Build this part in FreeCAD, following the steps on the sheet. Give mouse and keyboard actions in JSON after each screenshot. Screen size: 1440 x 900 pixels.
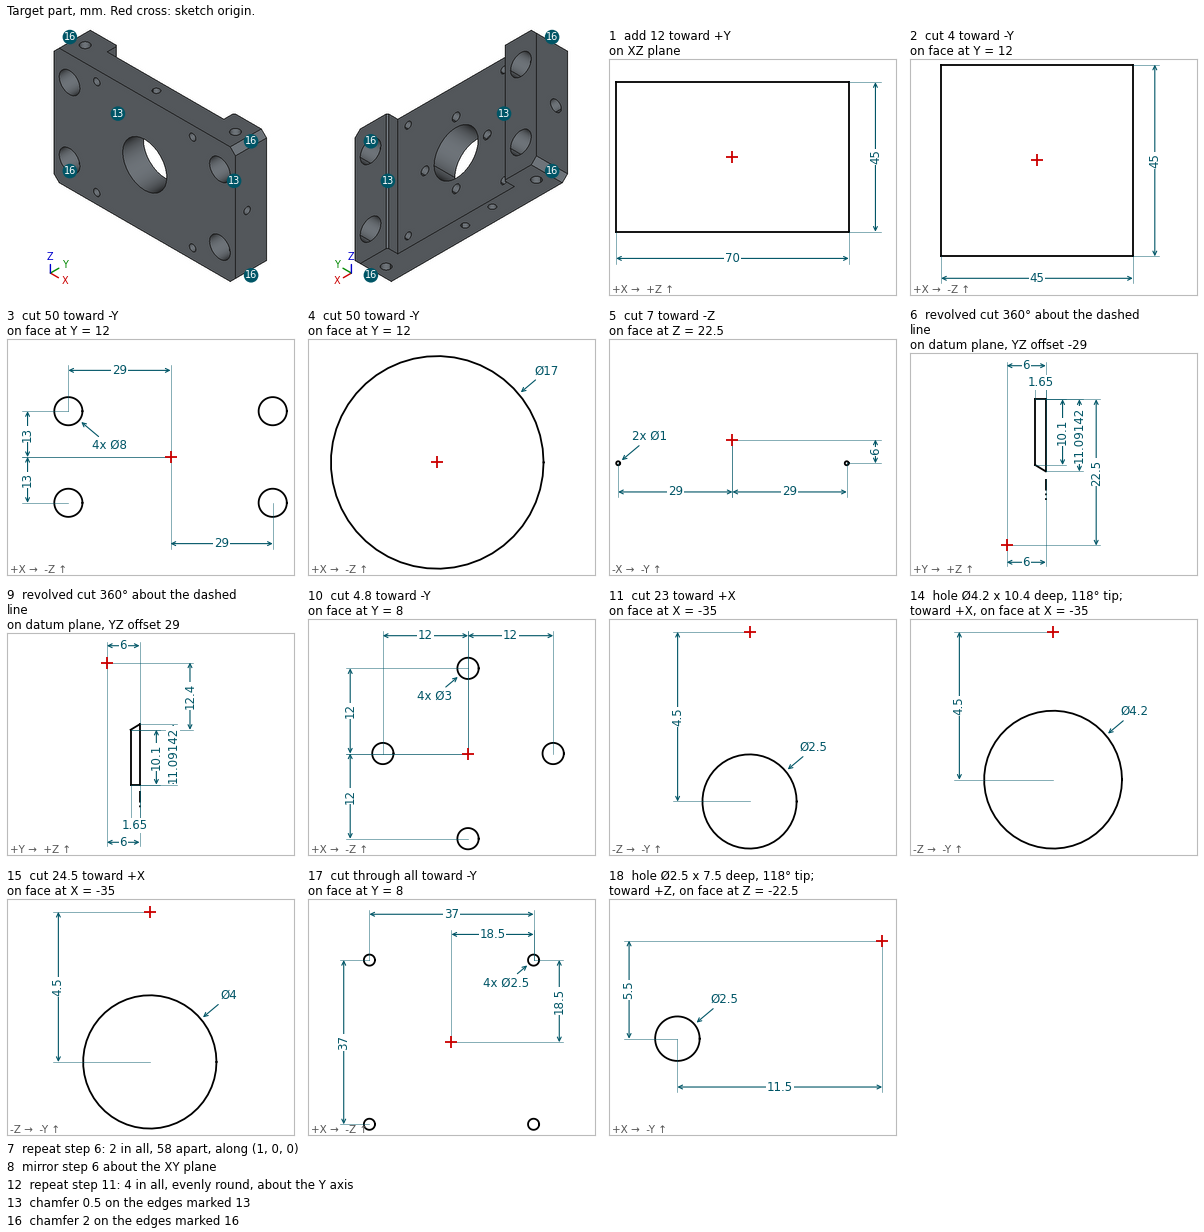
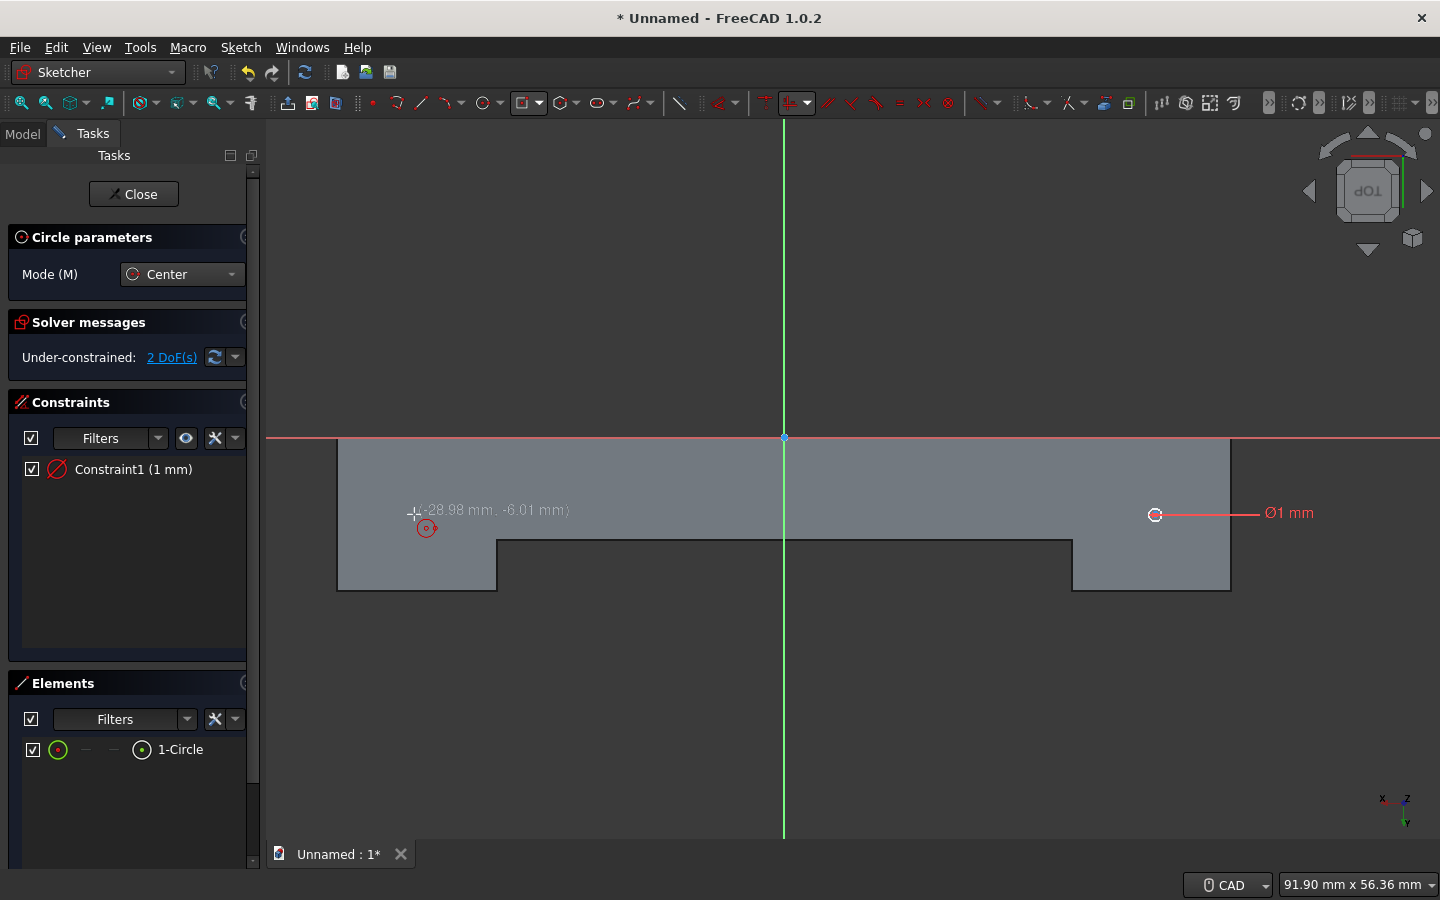
{"action": "left_click", "coordinate": [414, 514]}
{"action": "mouse_move", "coordinate": [418, 510]}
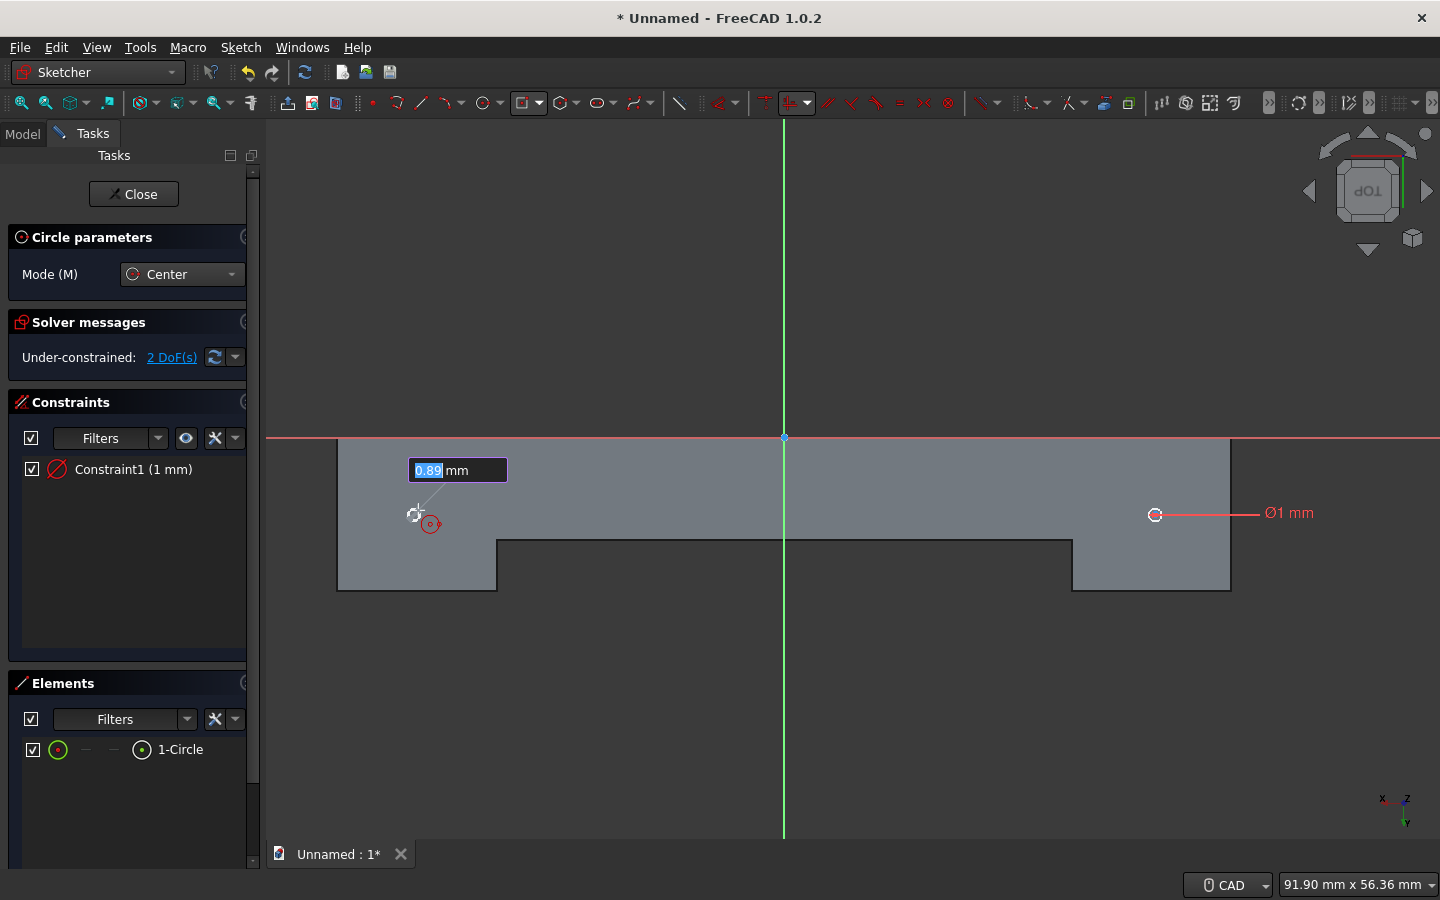
{"action": "type", "text": "1"}
{"action": "key", "text": "Return"}
{"action": "key", "text": "Escape"}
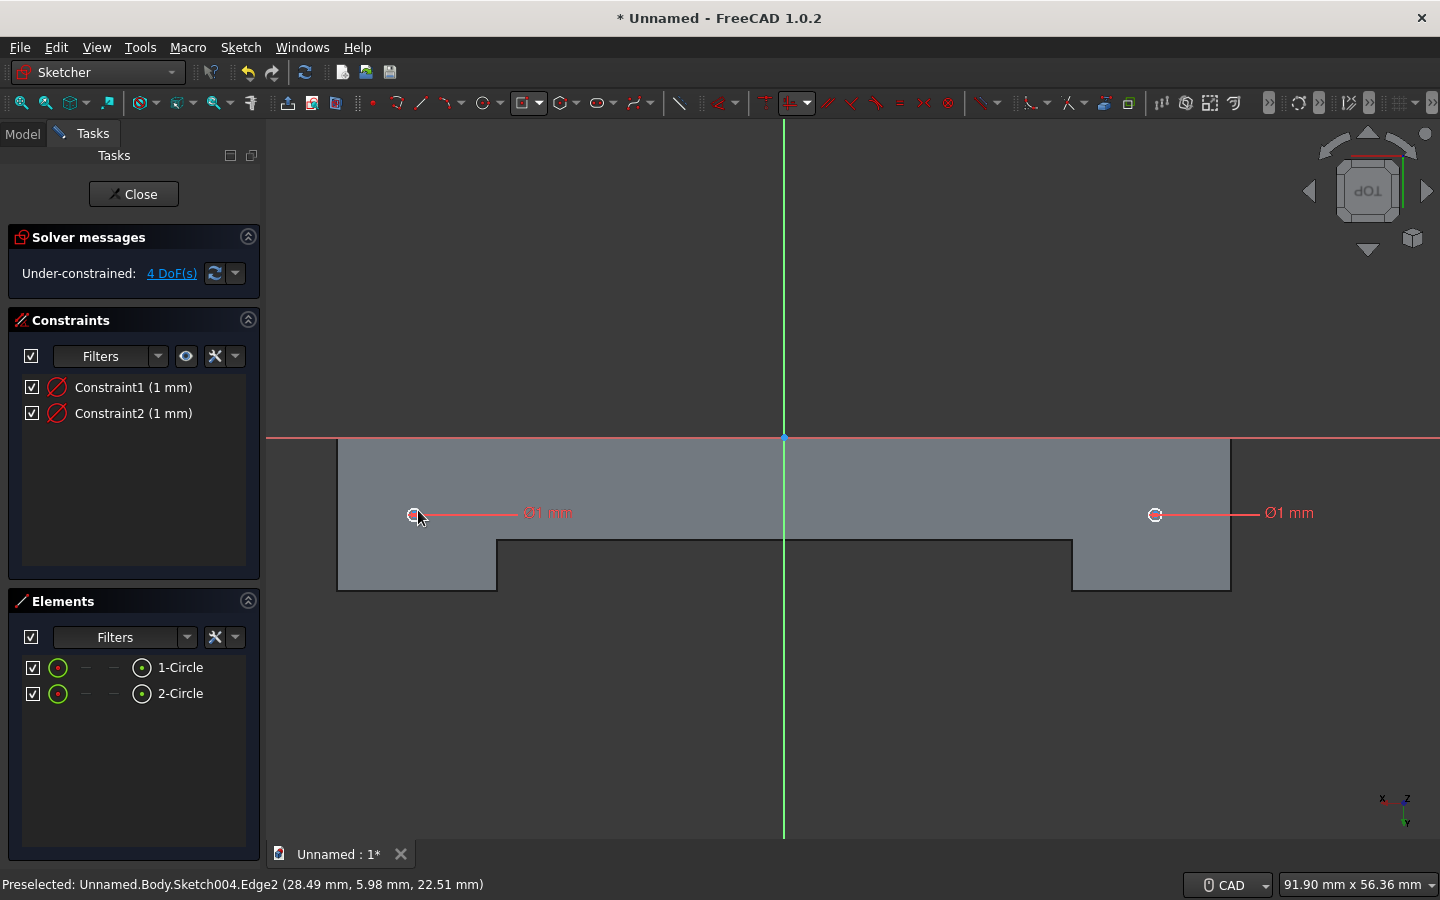
{"action": "left_click", "coordinate": [1155, 515]}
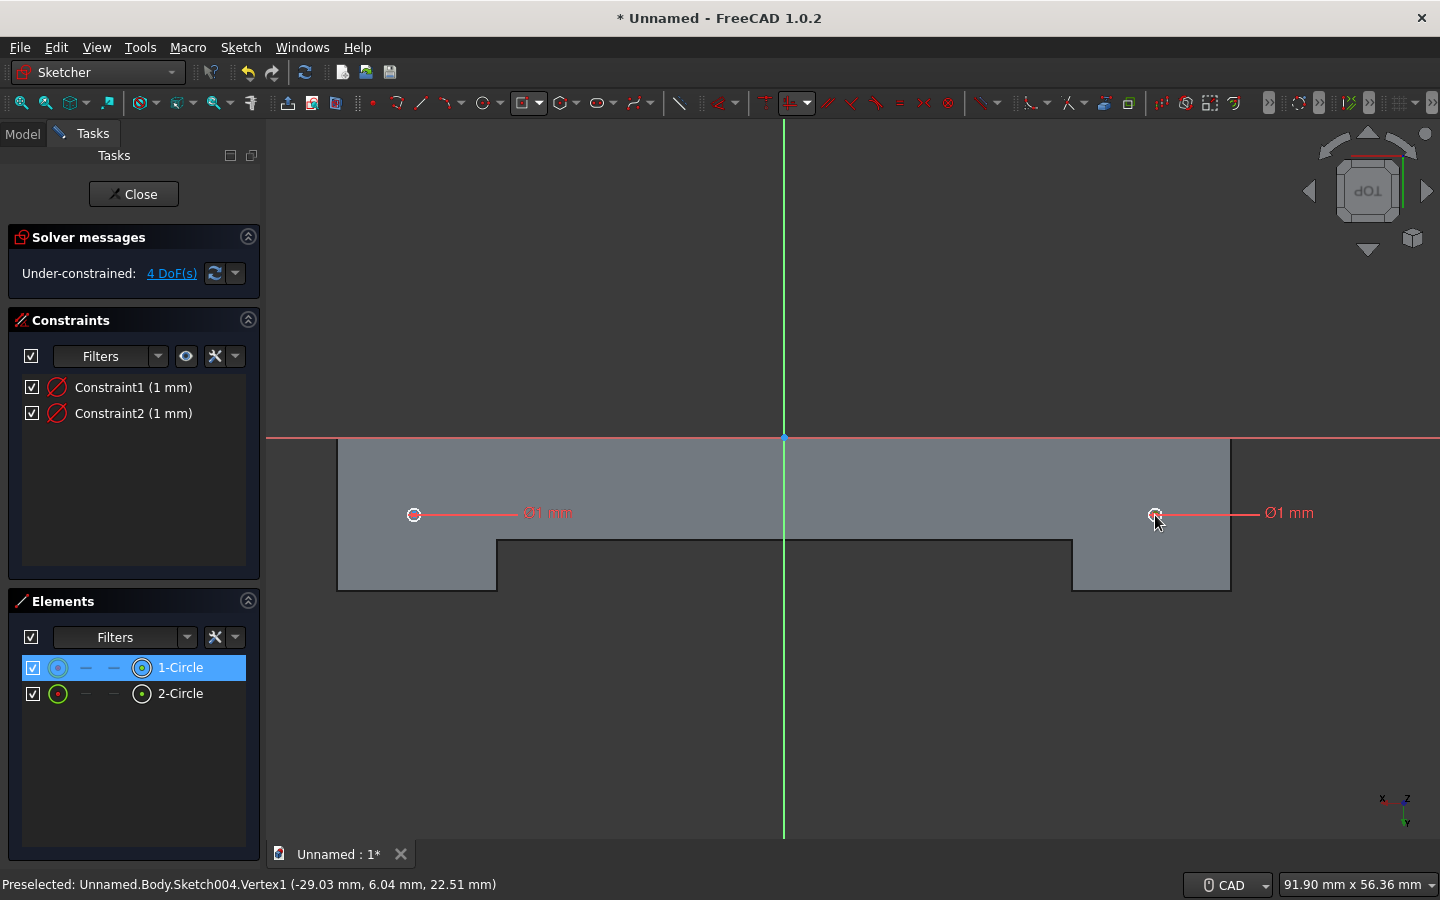
{"action": "left_click", "coordinate": [414, 515]}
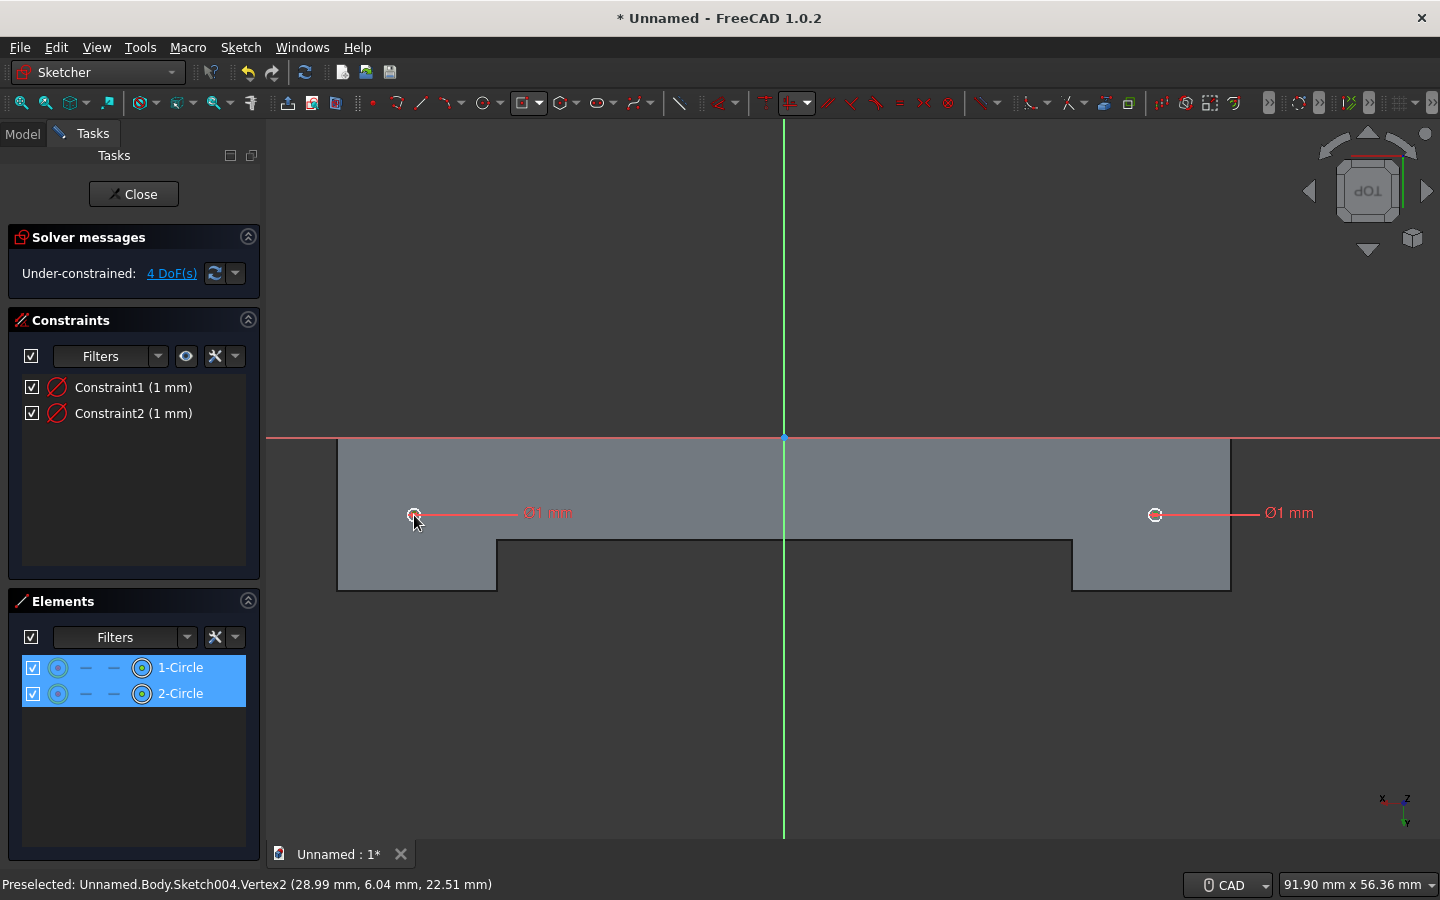
{"action": "left_click", "coordinate": [810, 104]}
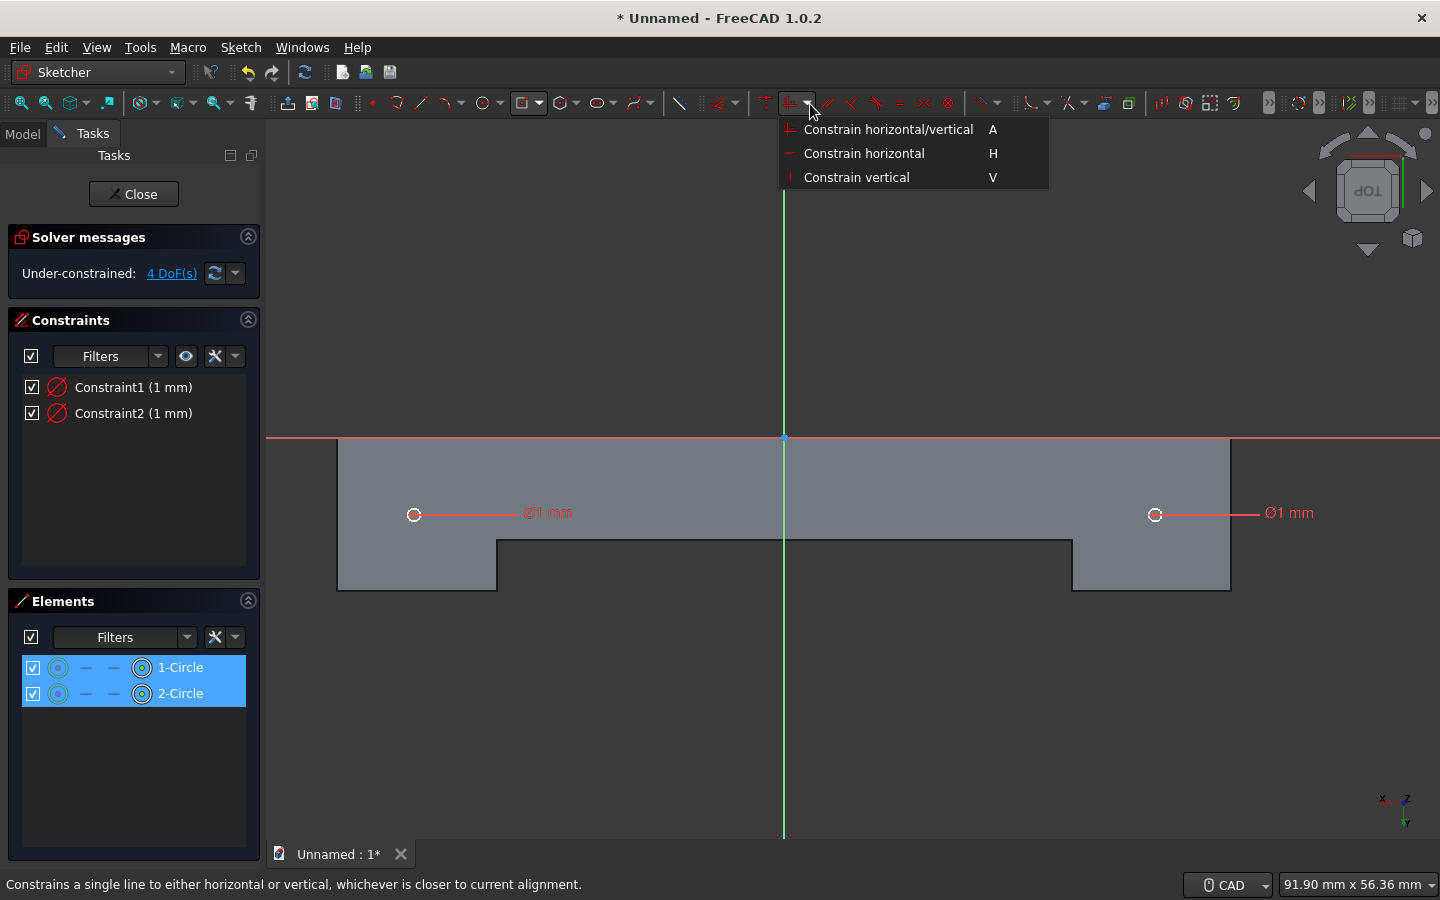
{"action": "left_click", "coordinate": [914, 153]}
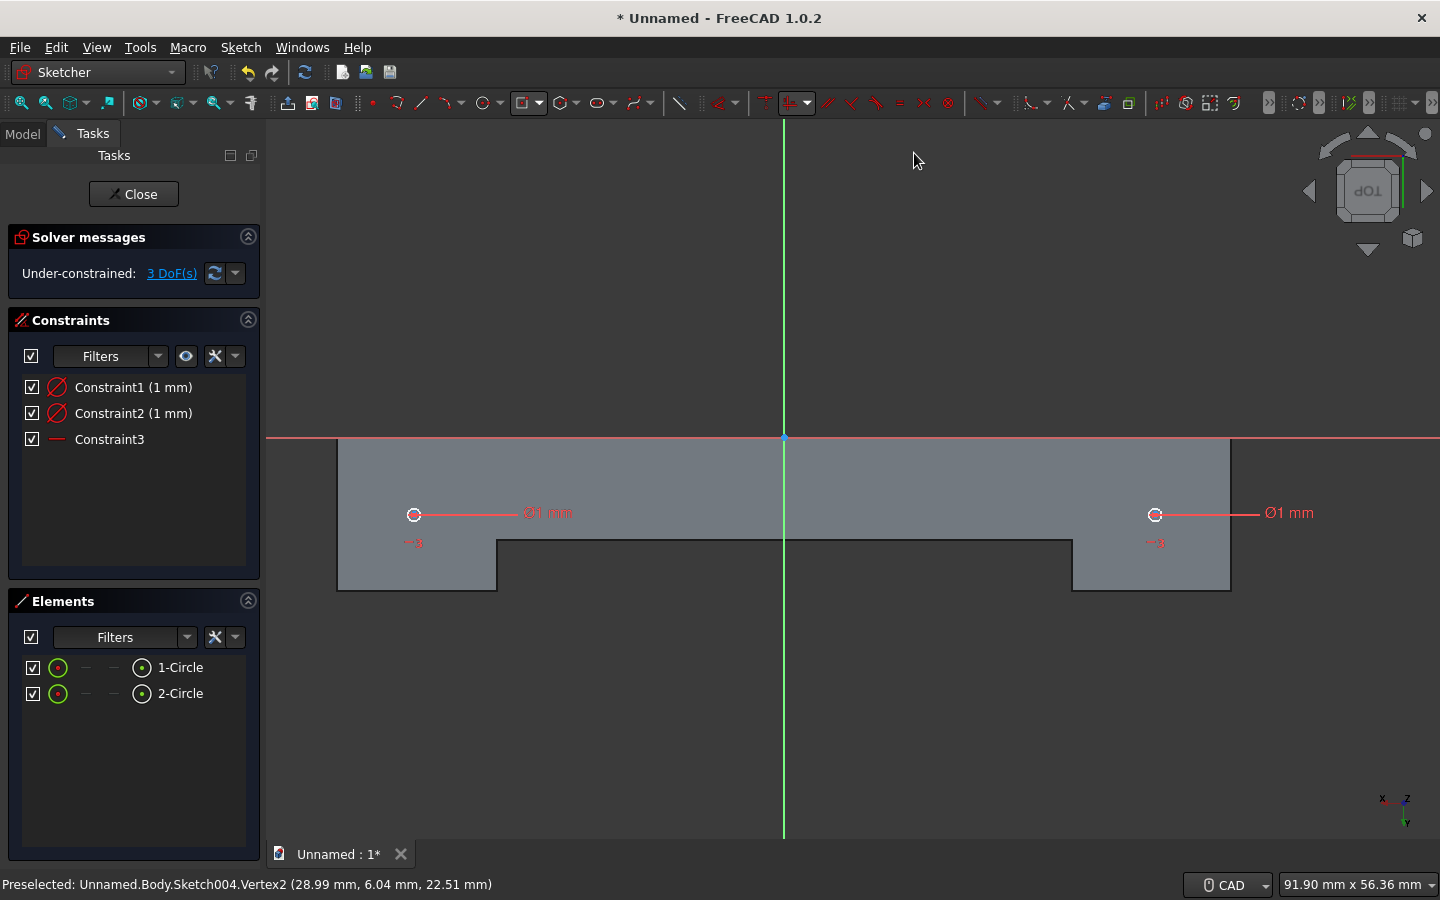
{"action": "left_click", "coordinate": [718, 104]}